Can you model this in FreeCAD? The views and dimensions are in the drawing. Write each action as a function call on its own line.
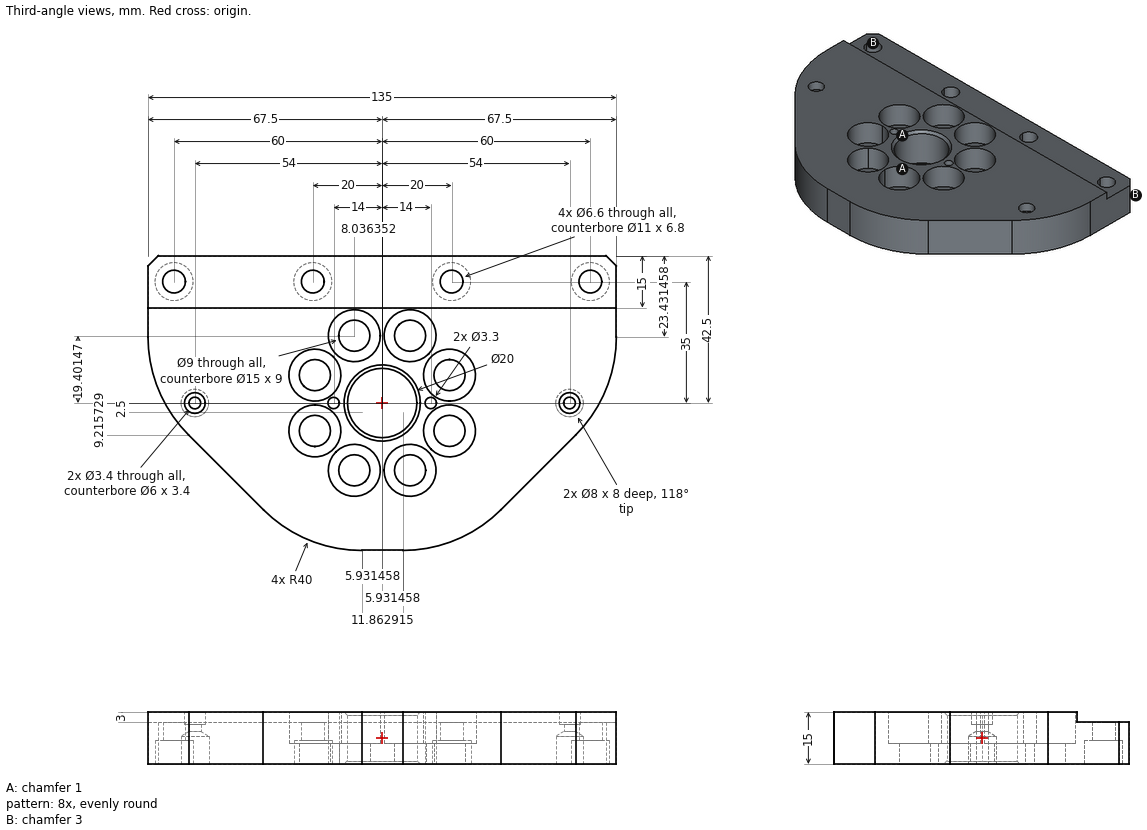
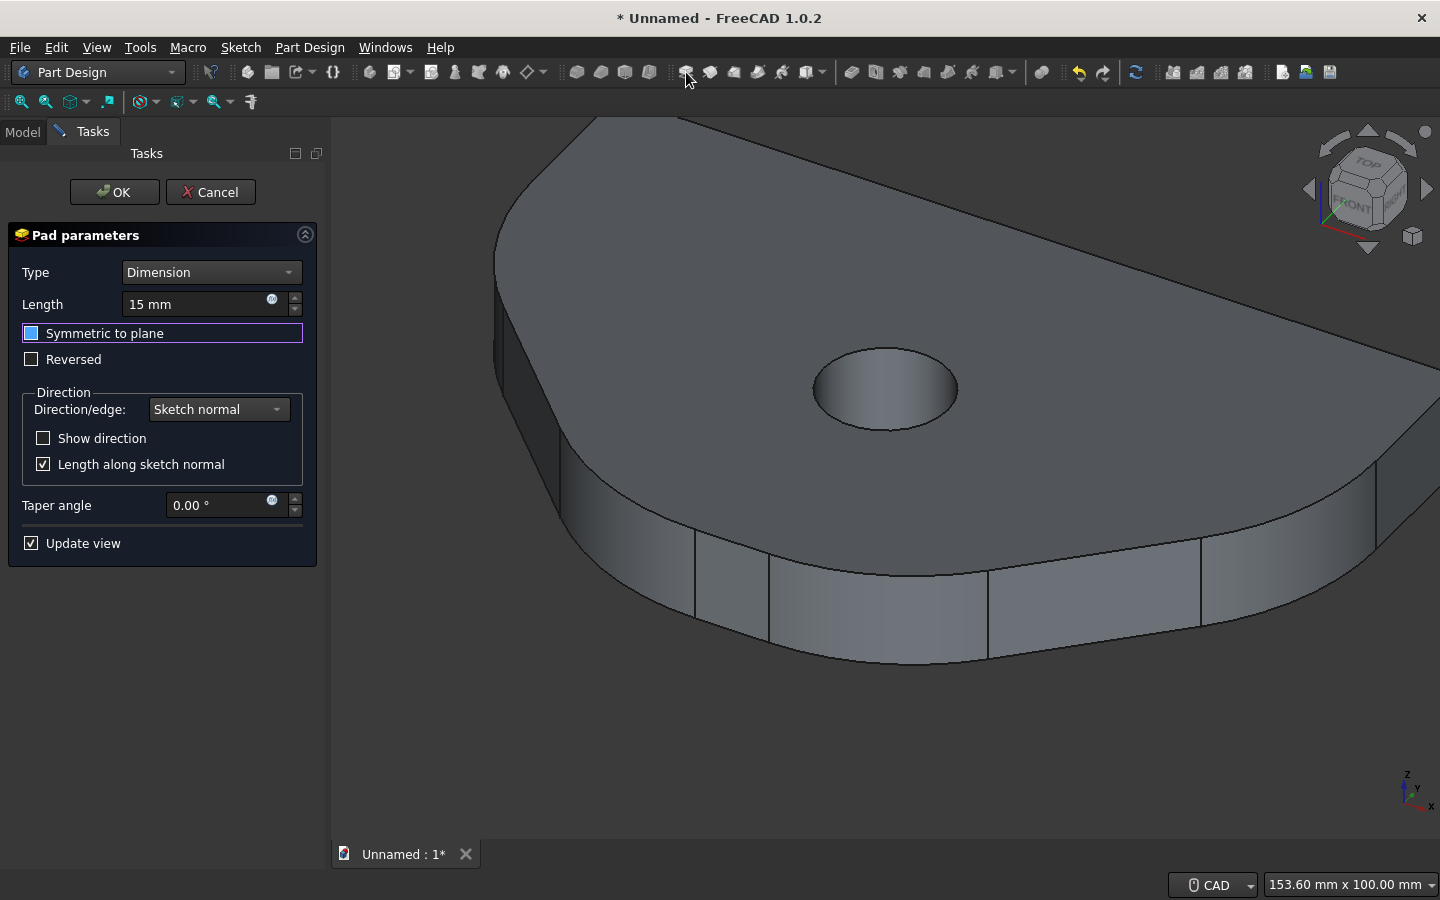
click(30, 333)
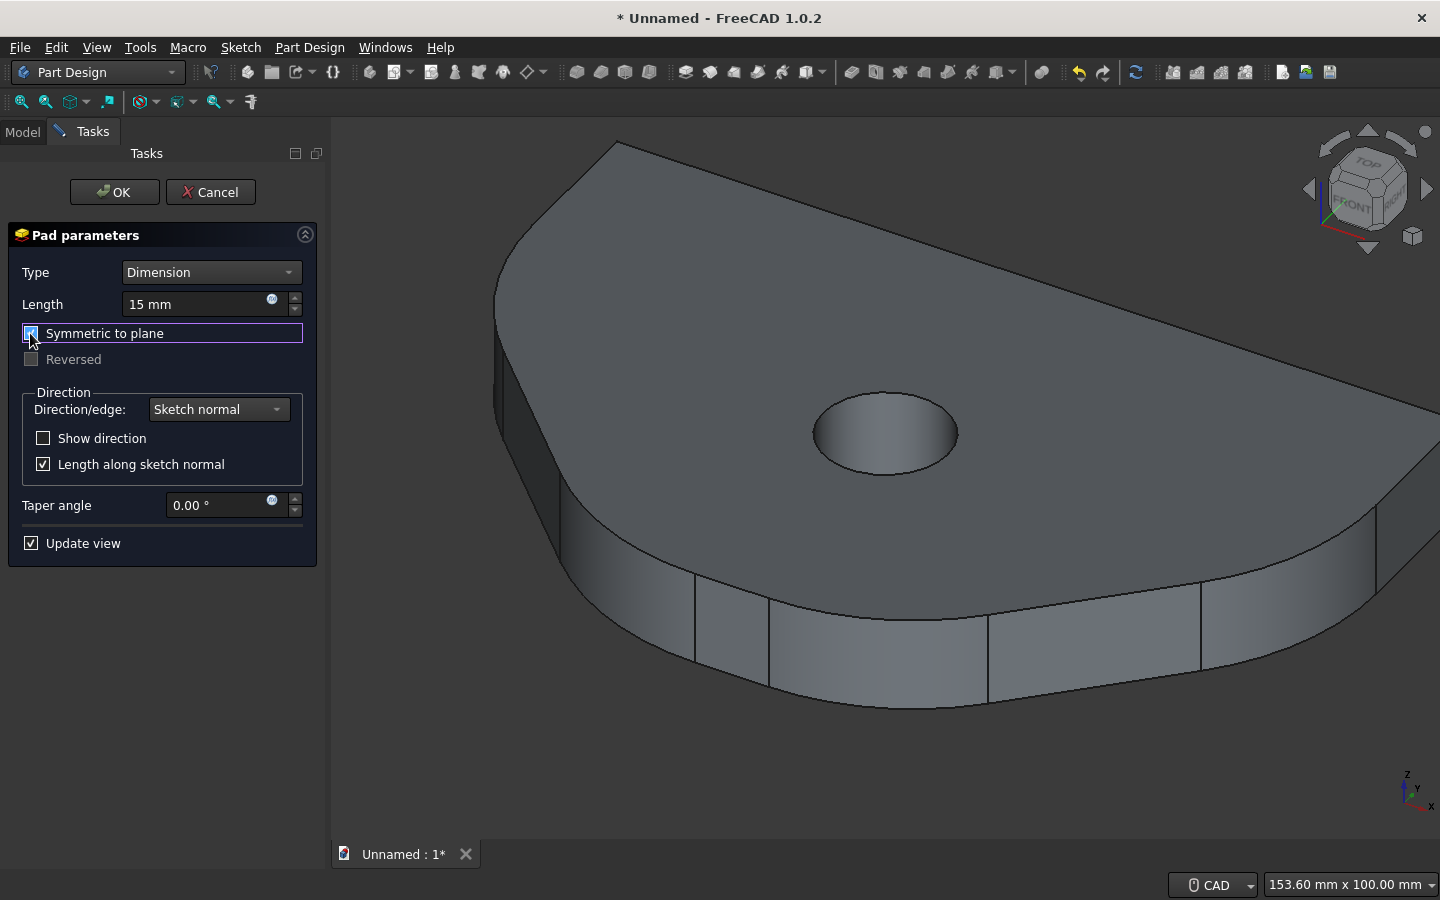
click(115, 192)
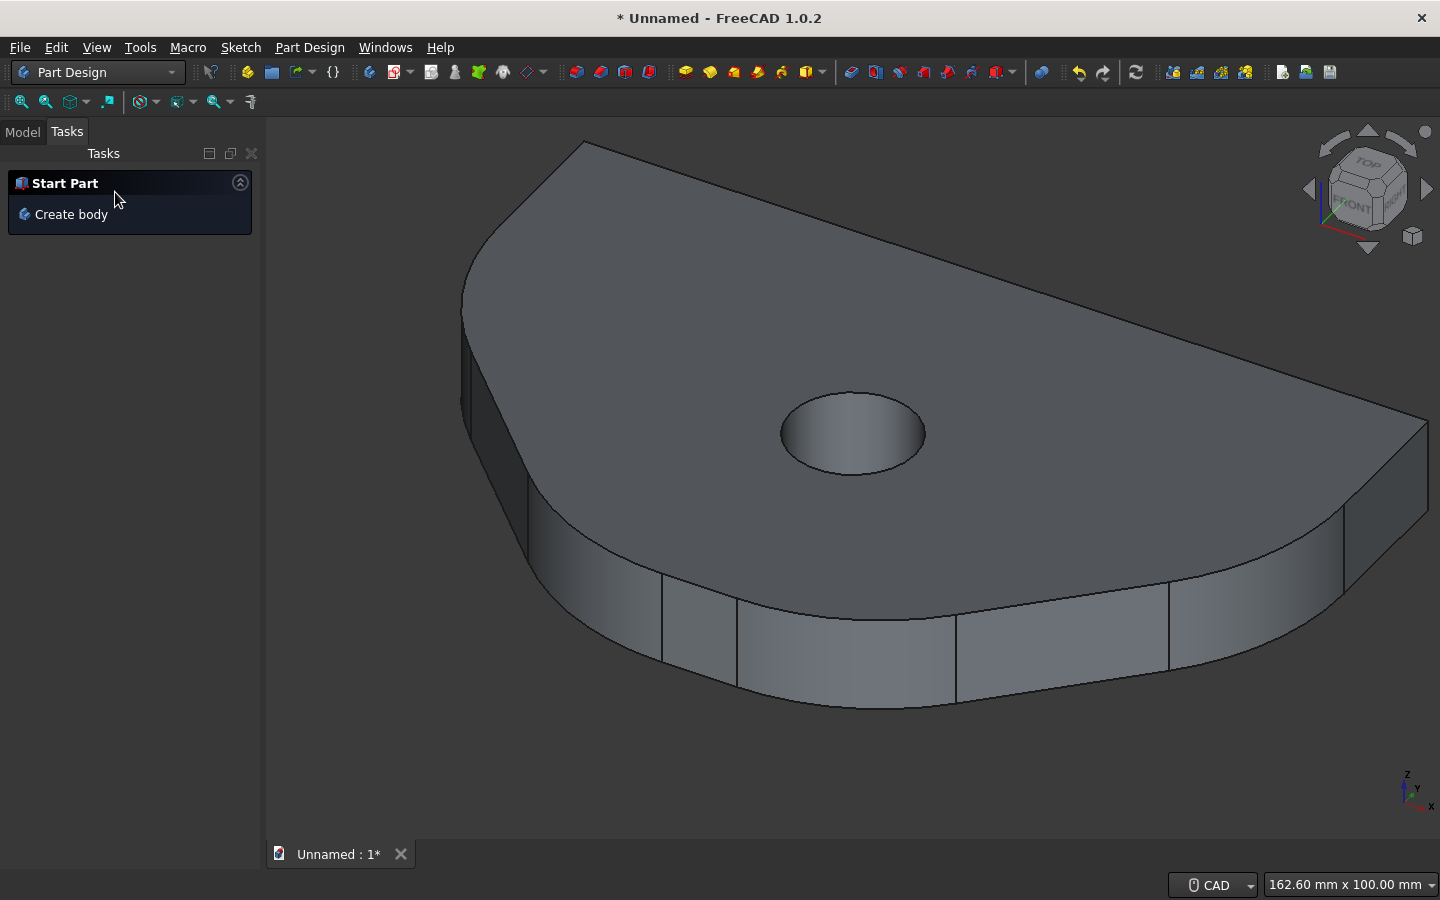
click(1138, 469)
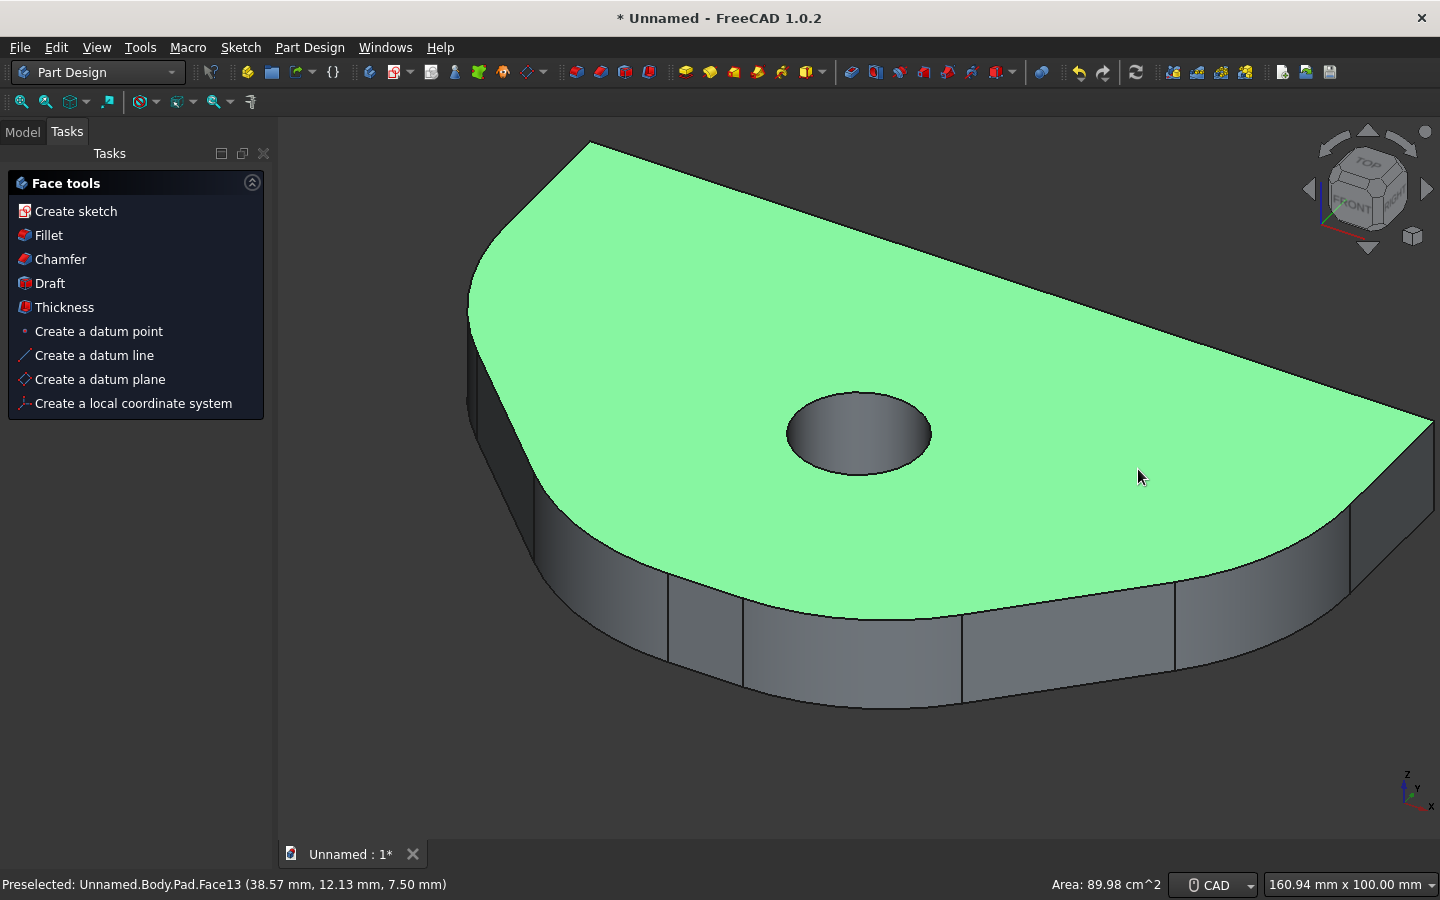
click(394, 72)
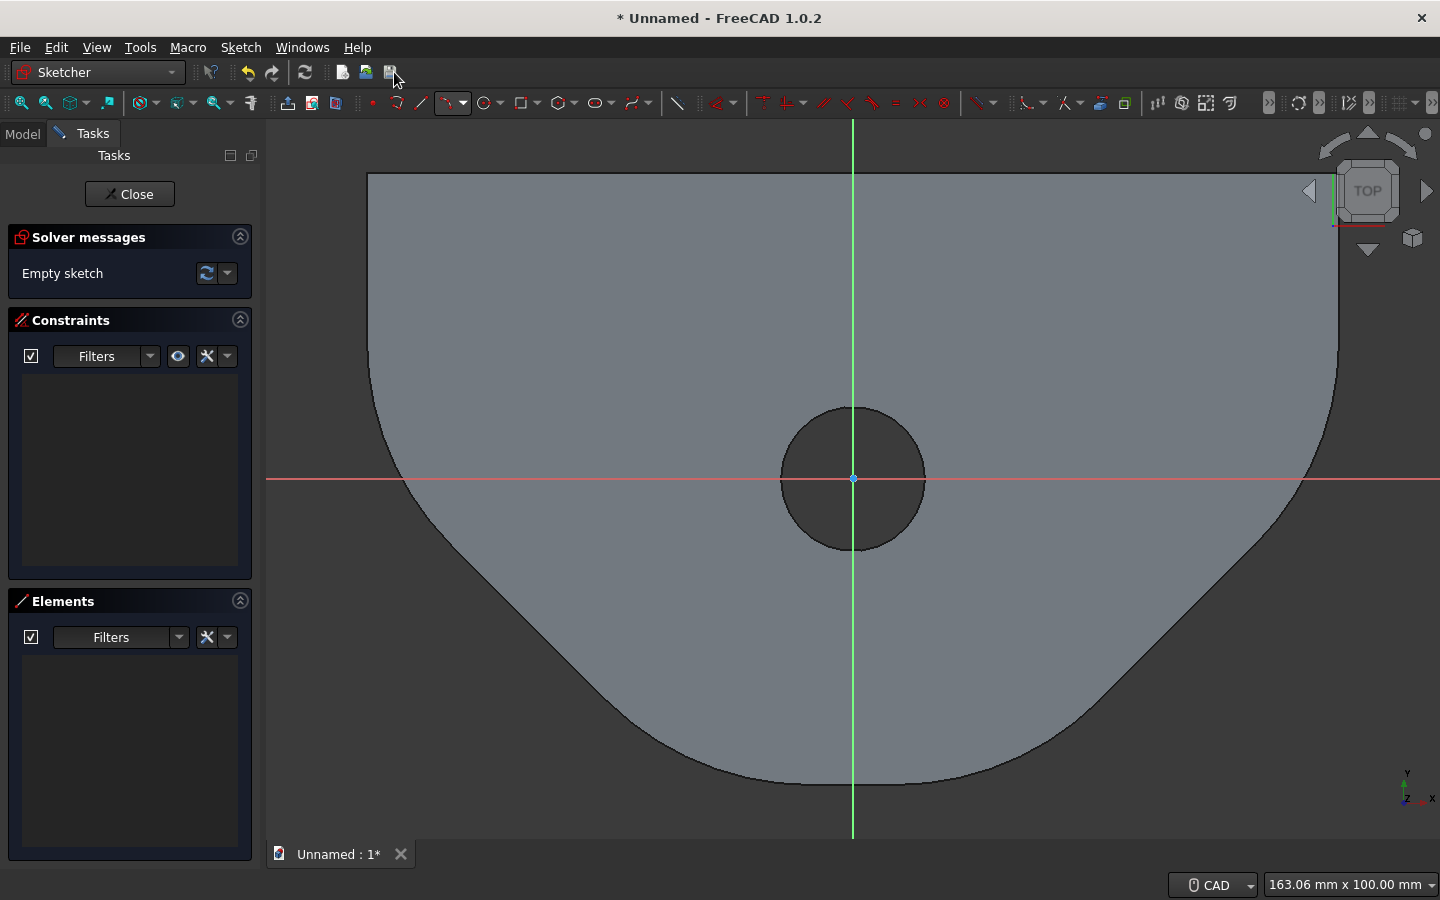
scroll(797, 317, up, 10)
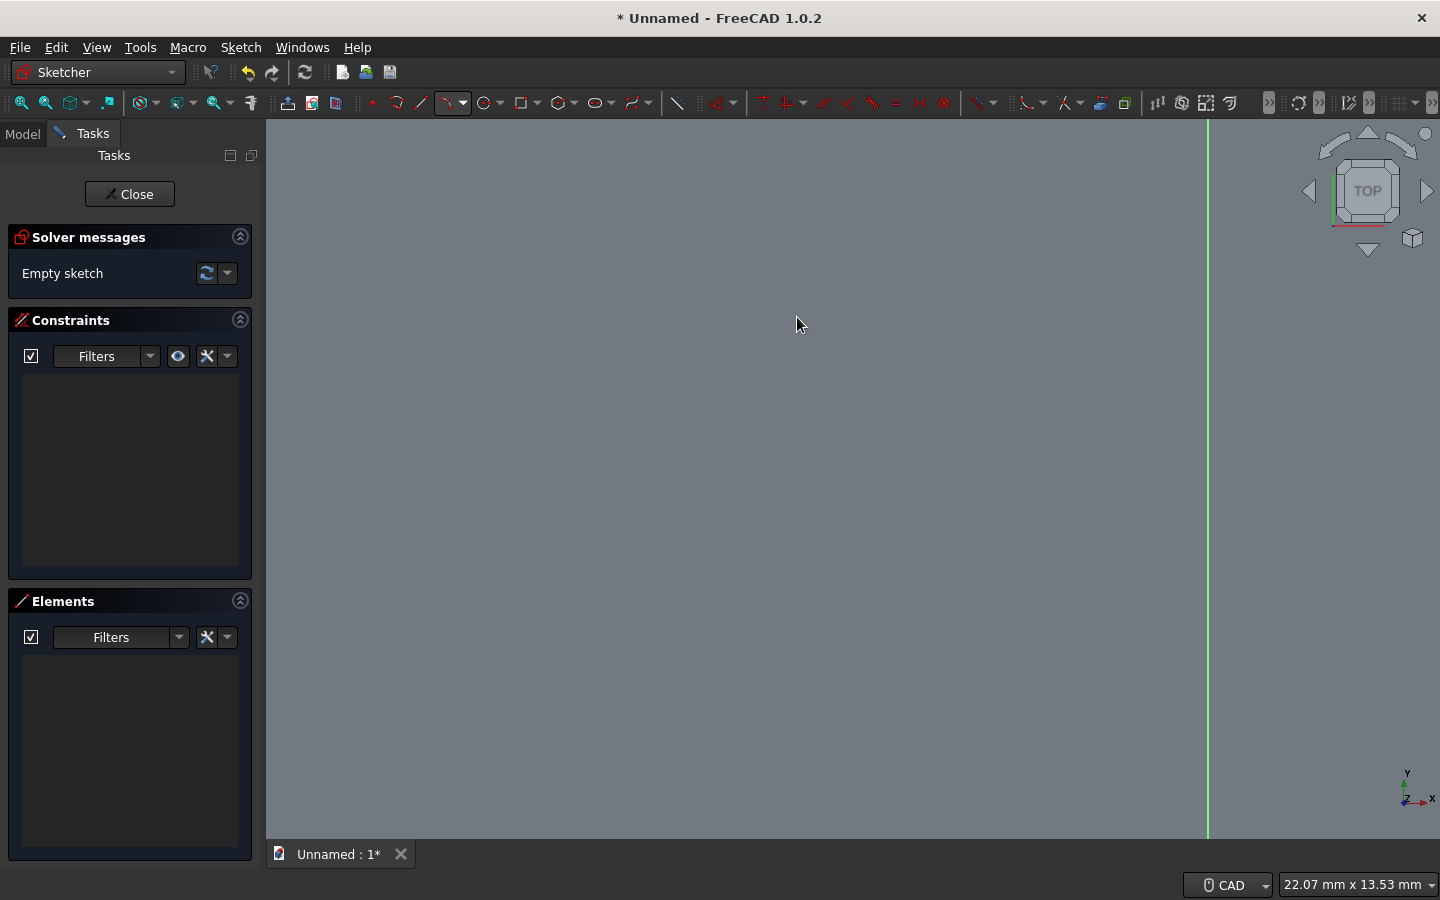
click(484, 104)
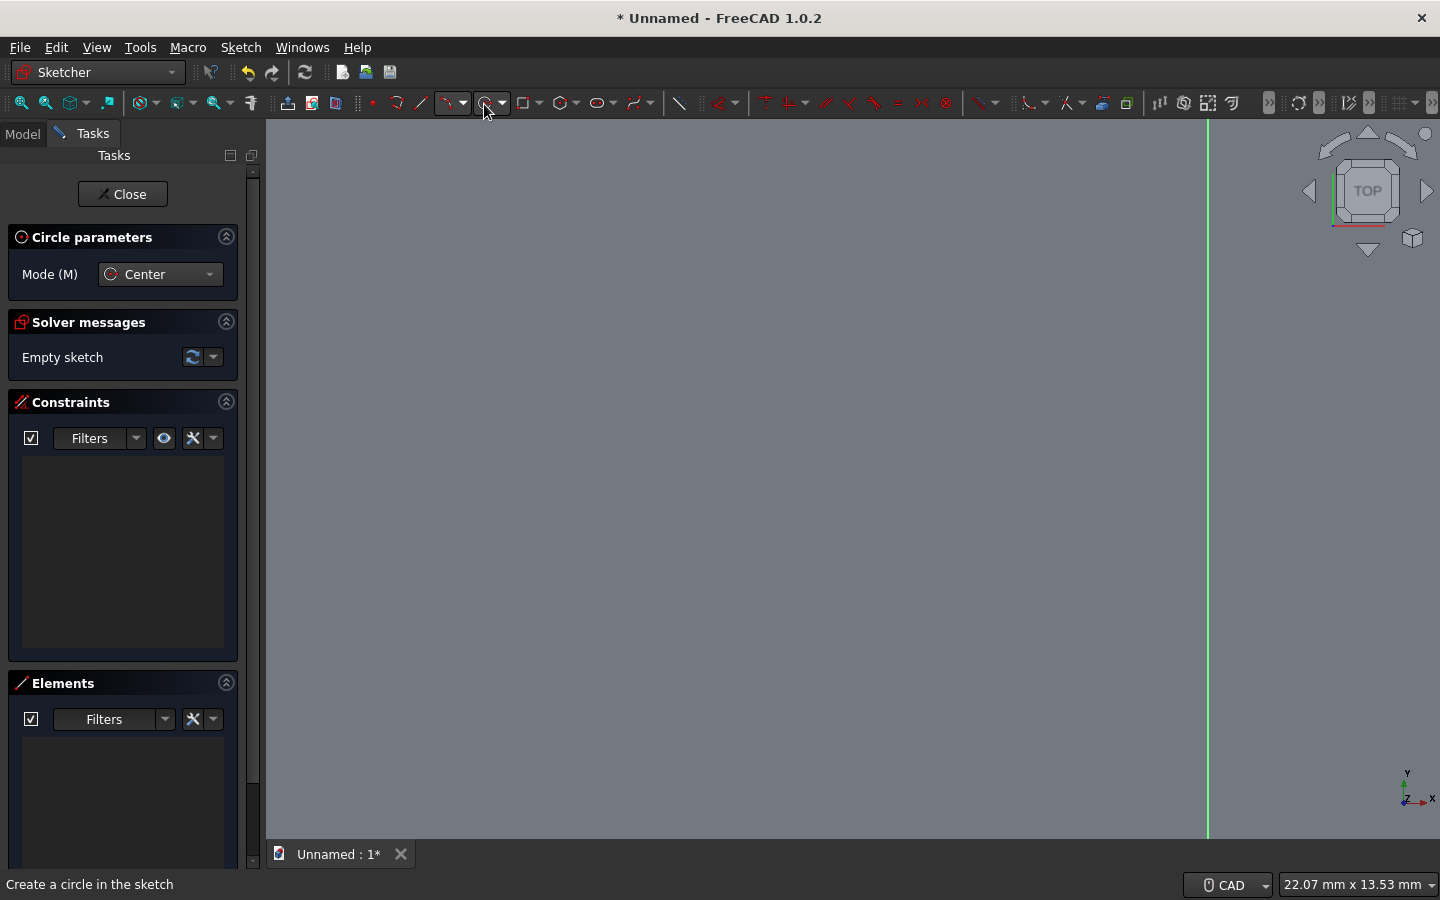
click(780, 480)
move(950, 311)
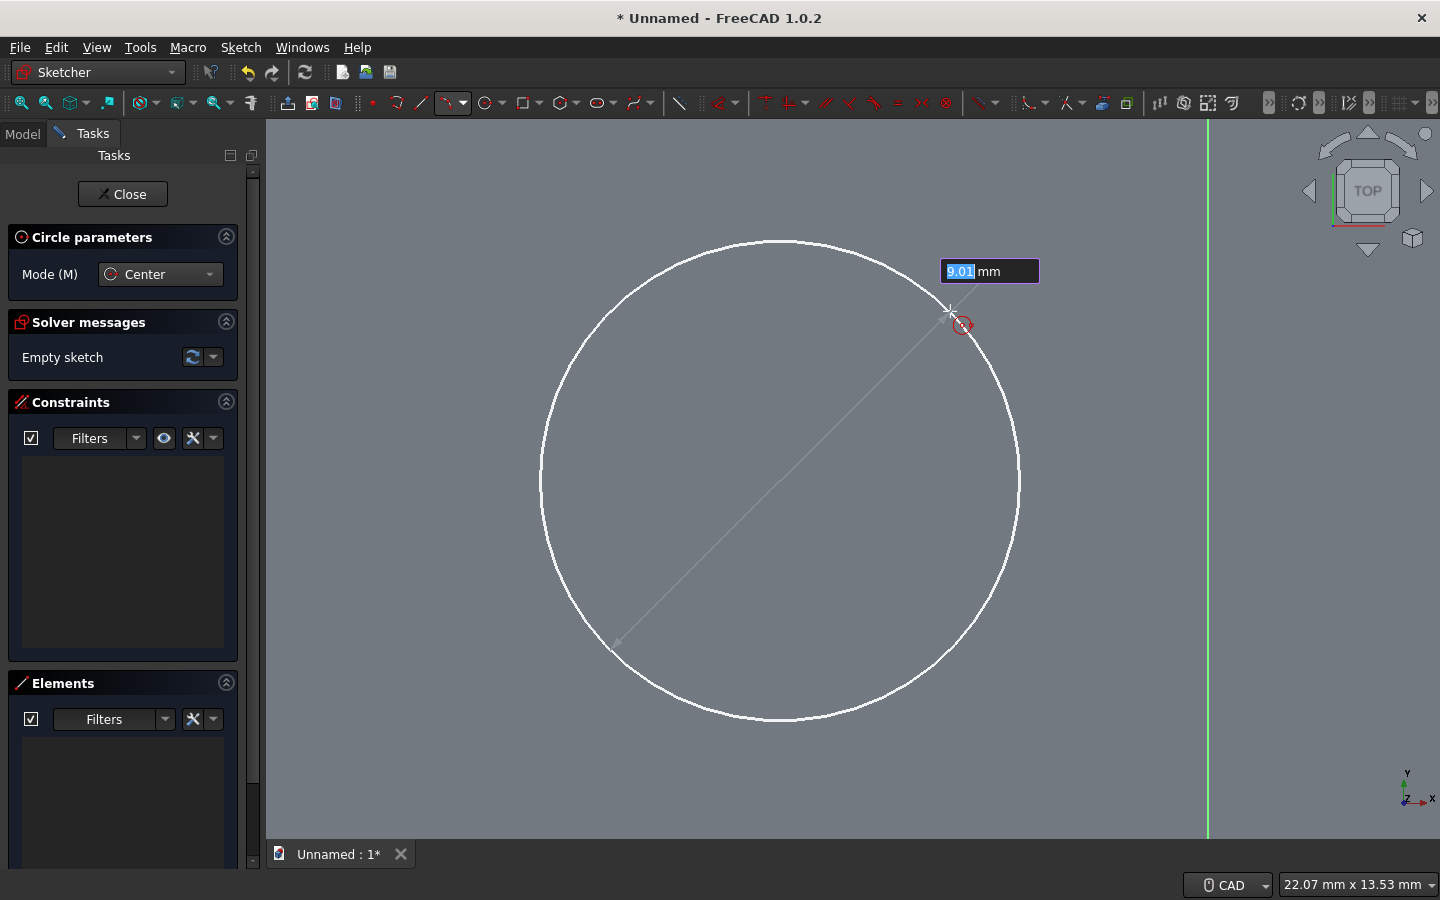
text(9)
key(Return)
key(Escape)